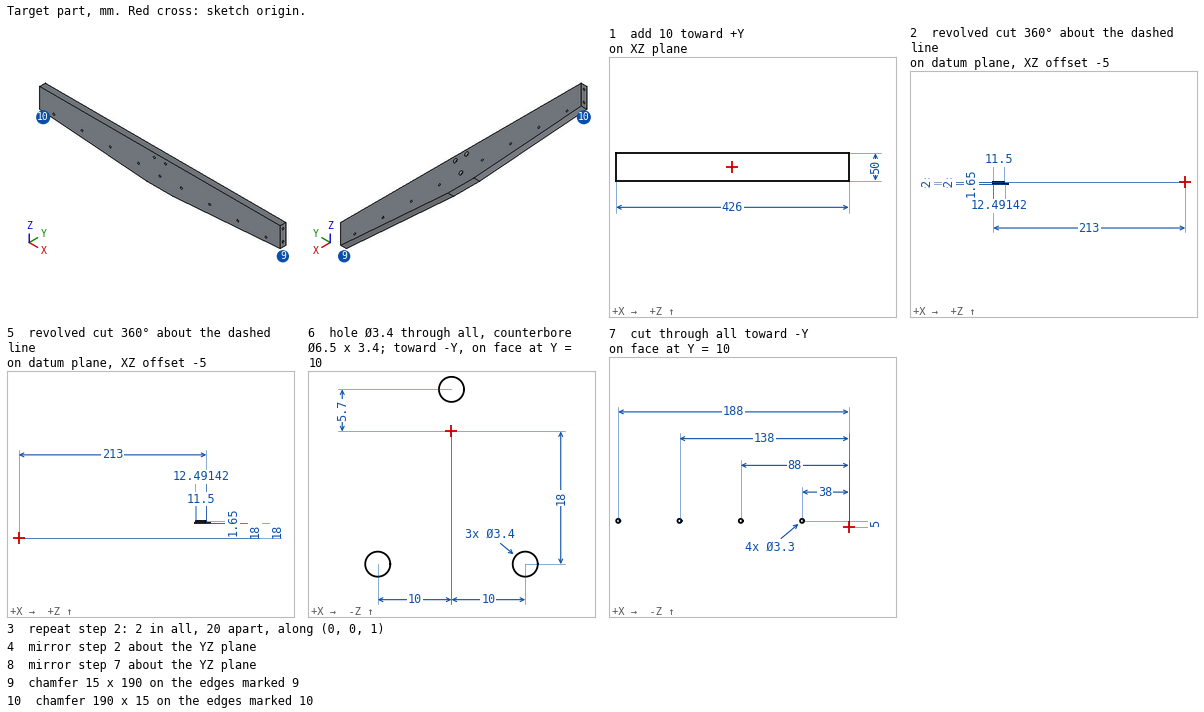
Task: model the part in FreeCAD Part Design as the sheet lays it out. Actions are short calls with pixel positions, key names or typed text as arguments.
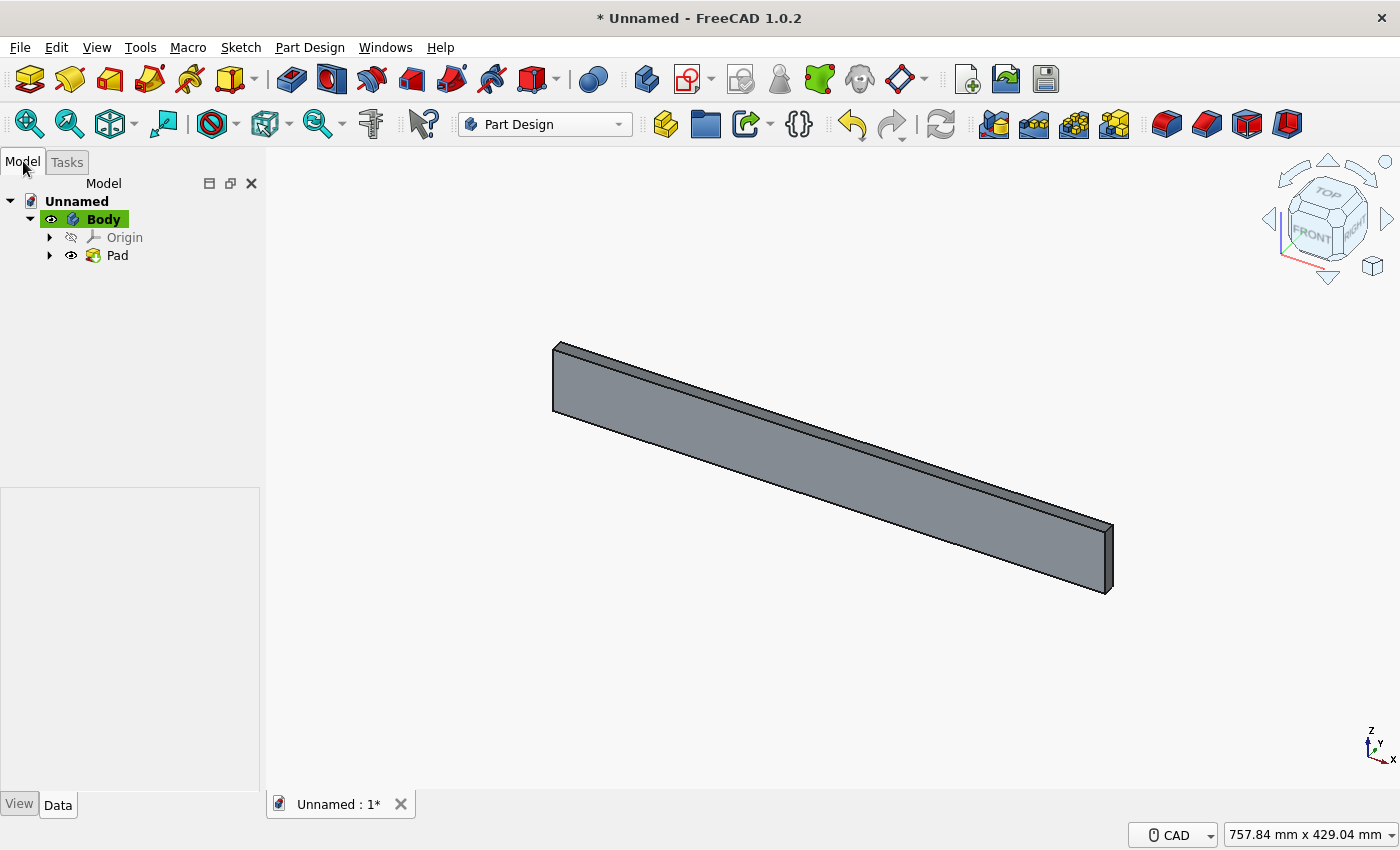
click(50, 237)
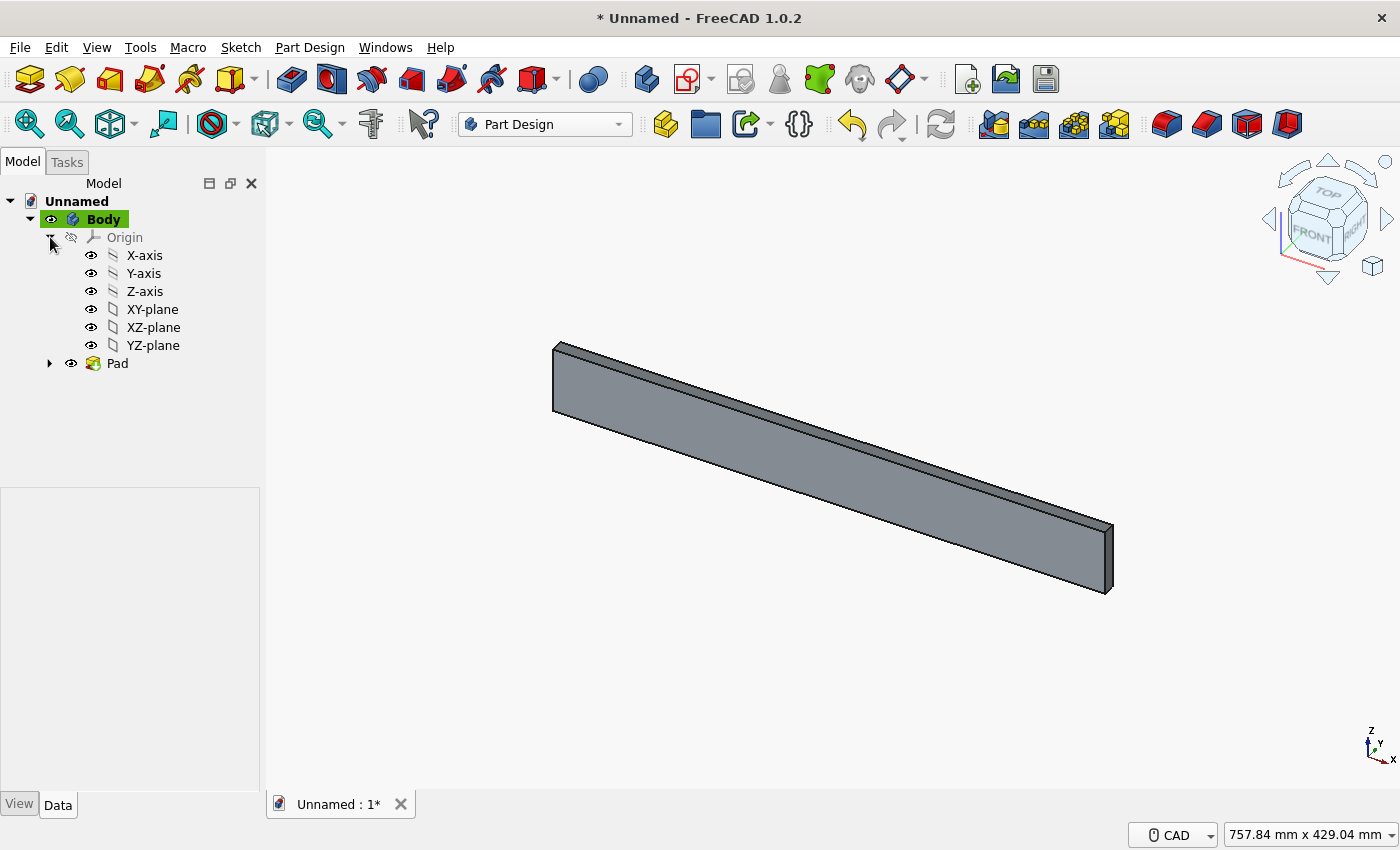
click(136, 327)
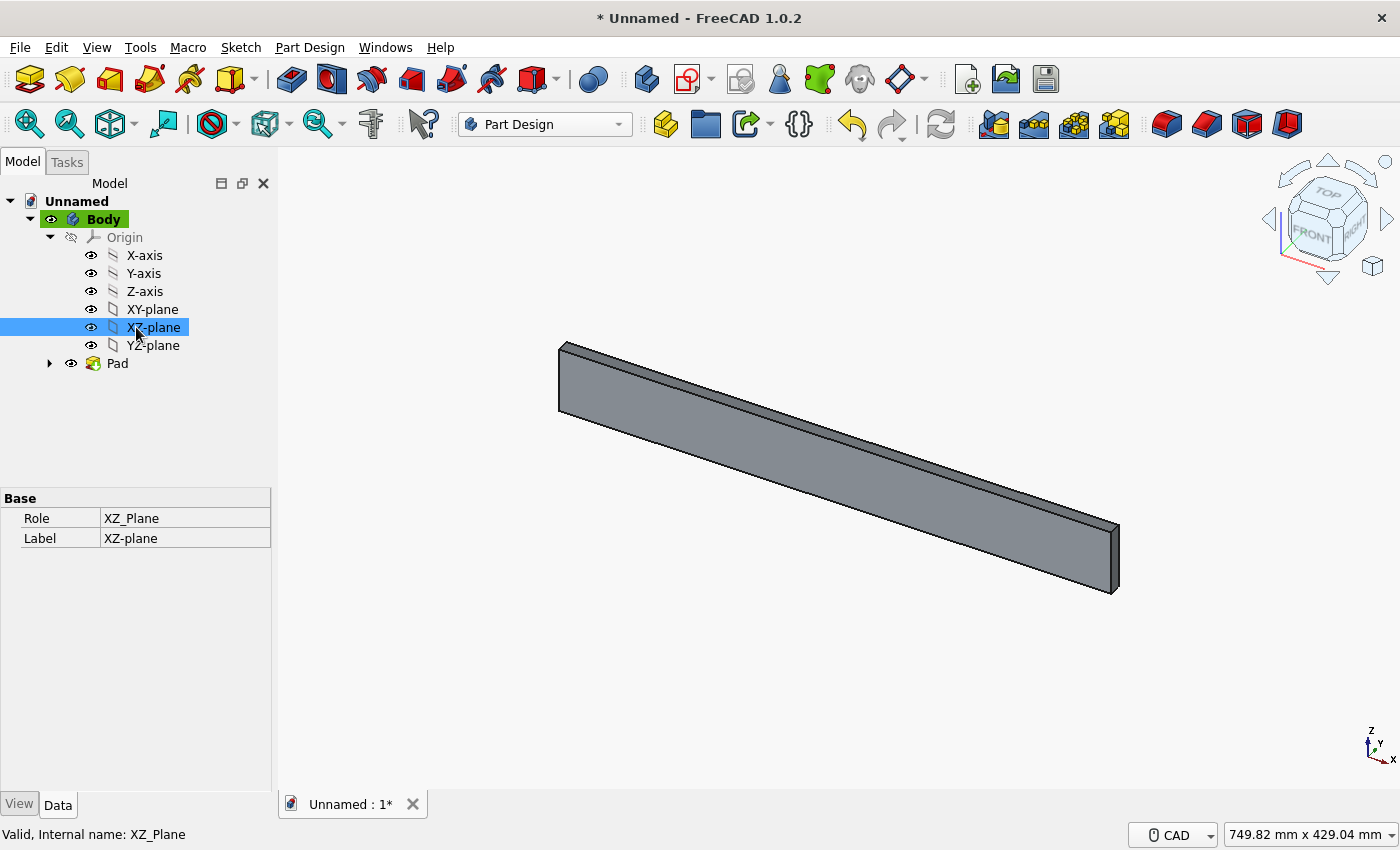
click(900, 80)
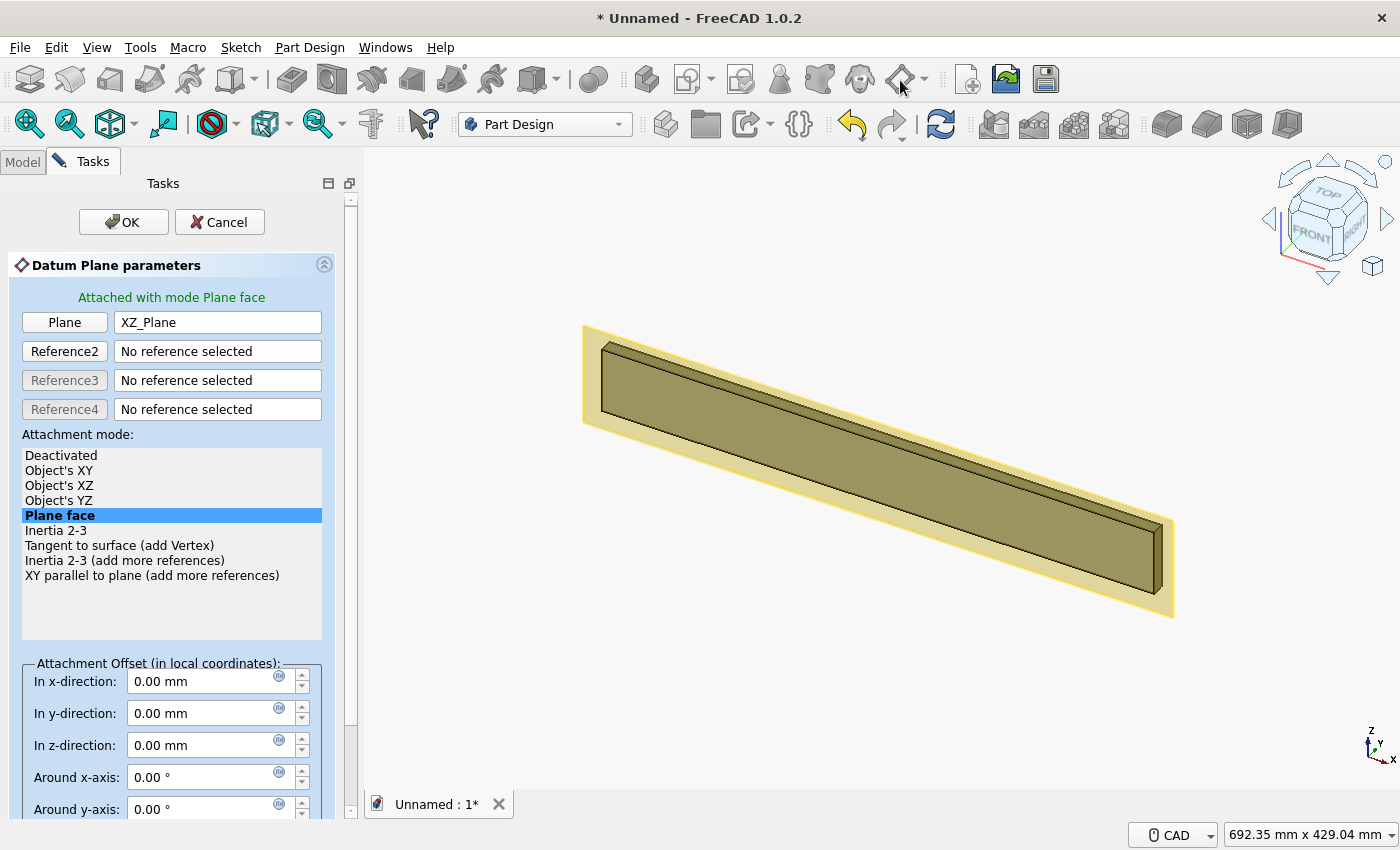
triple_click(210, 745)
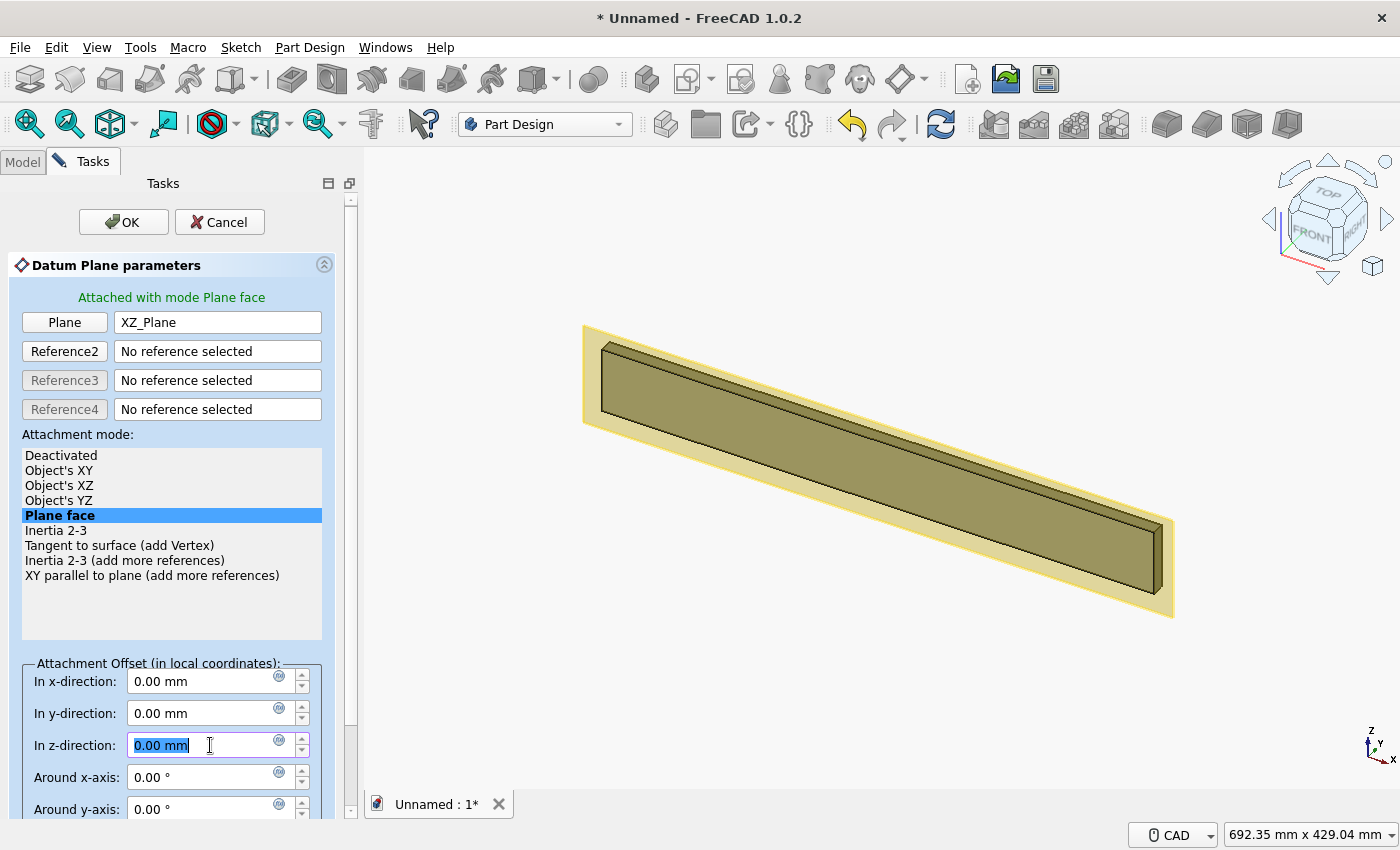
text(-5)
key(Tab)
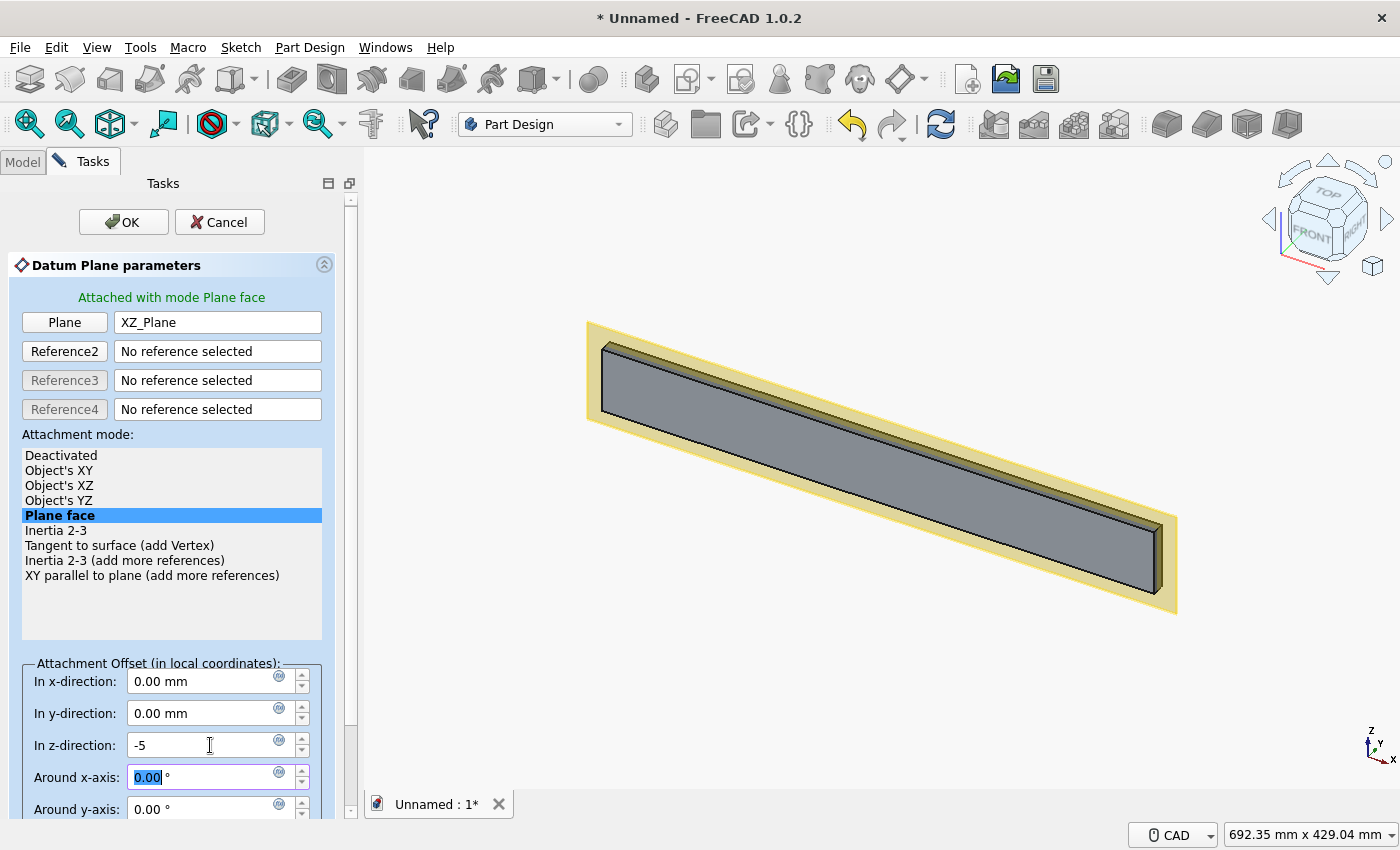
click(124, 222)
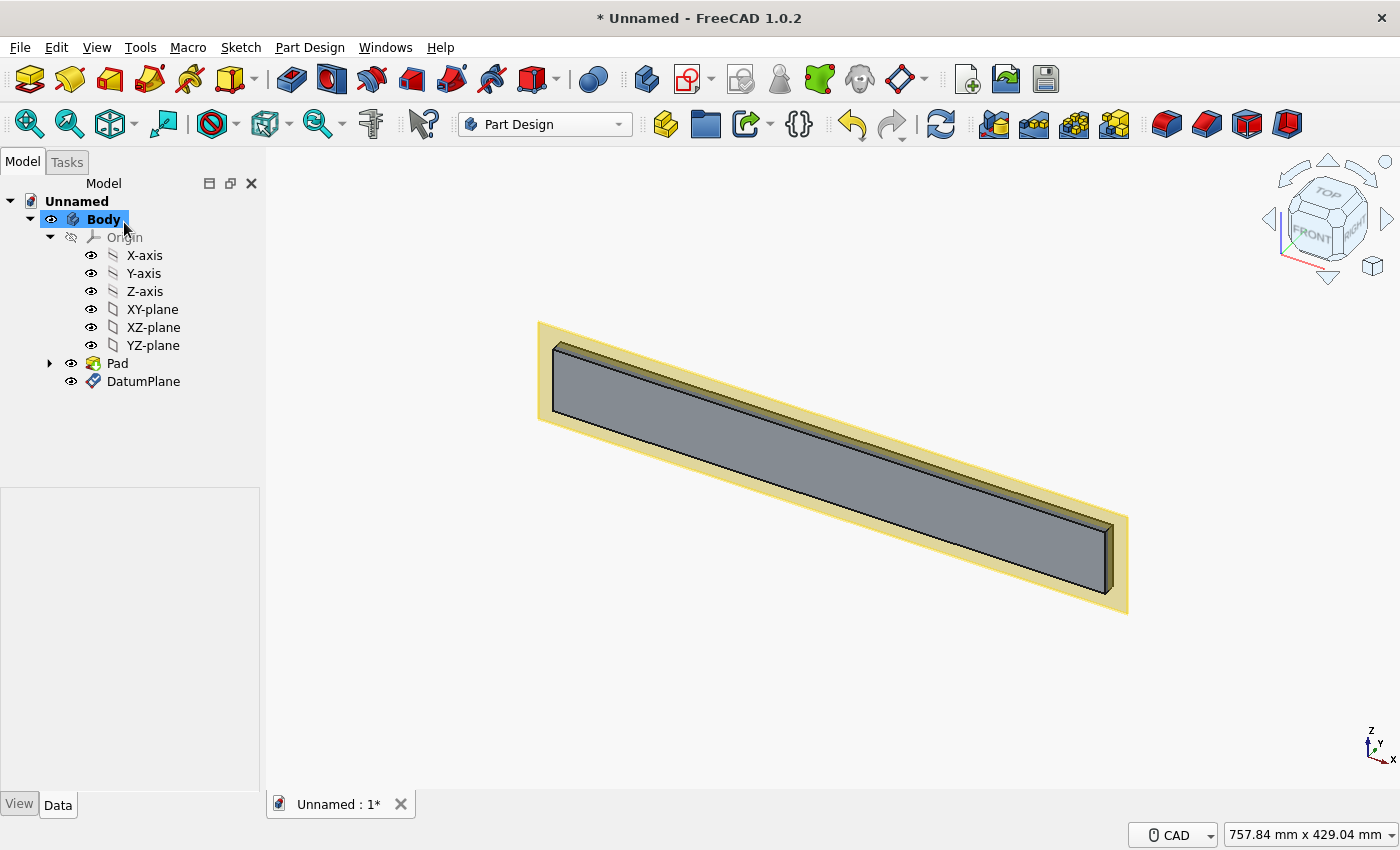
click(116, 381)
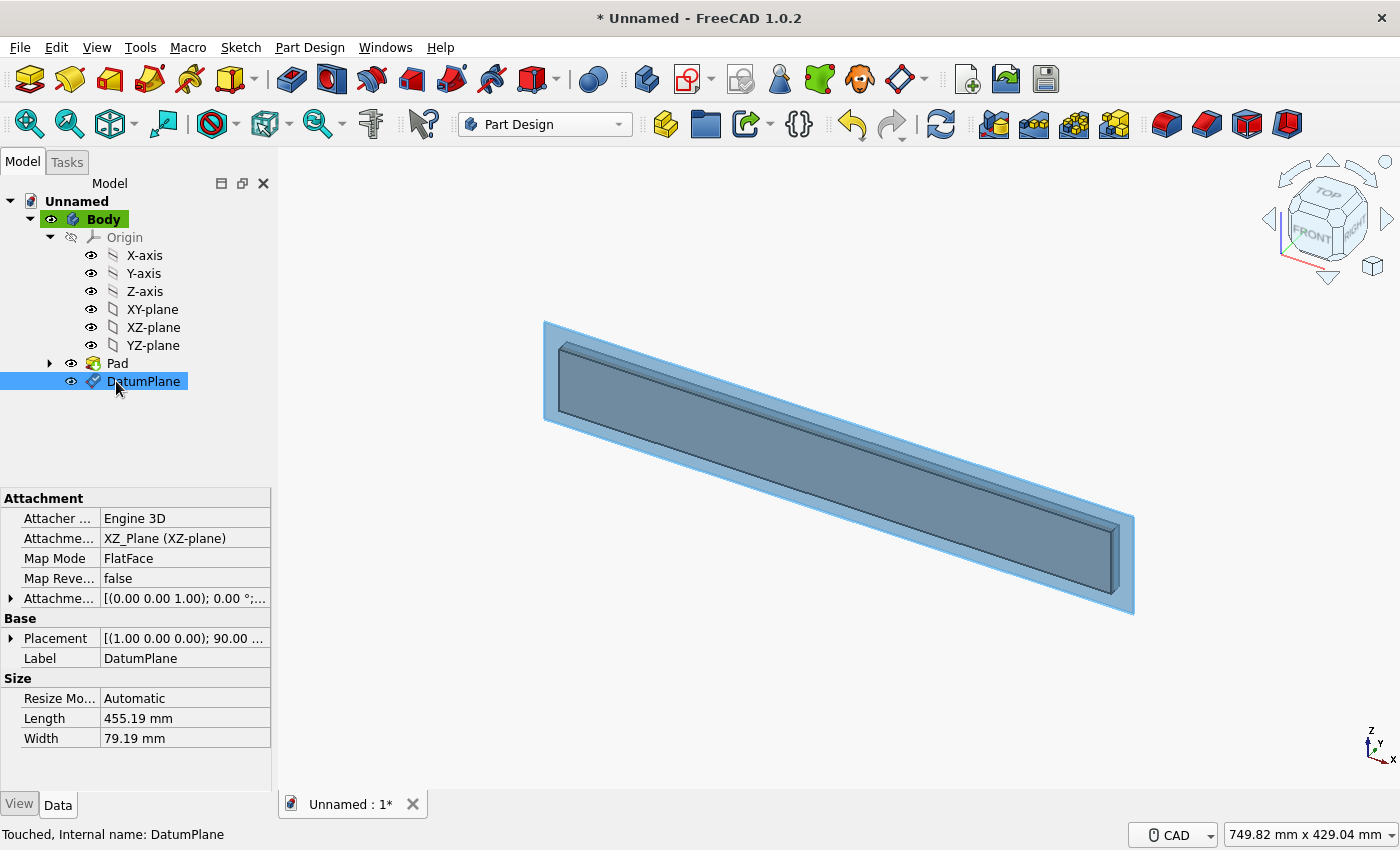
click(688, 80)